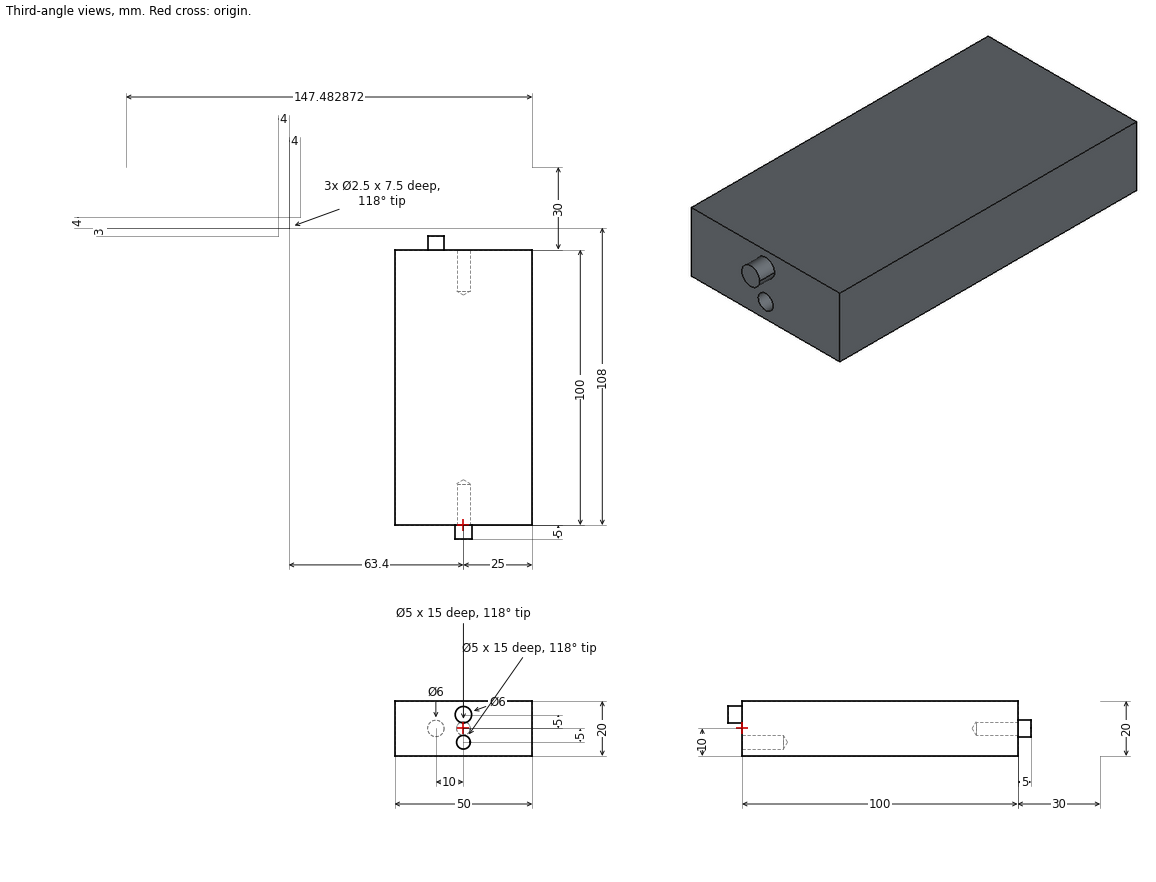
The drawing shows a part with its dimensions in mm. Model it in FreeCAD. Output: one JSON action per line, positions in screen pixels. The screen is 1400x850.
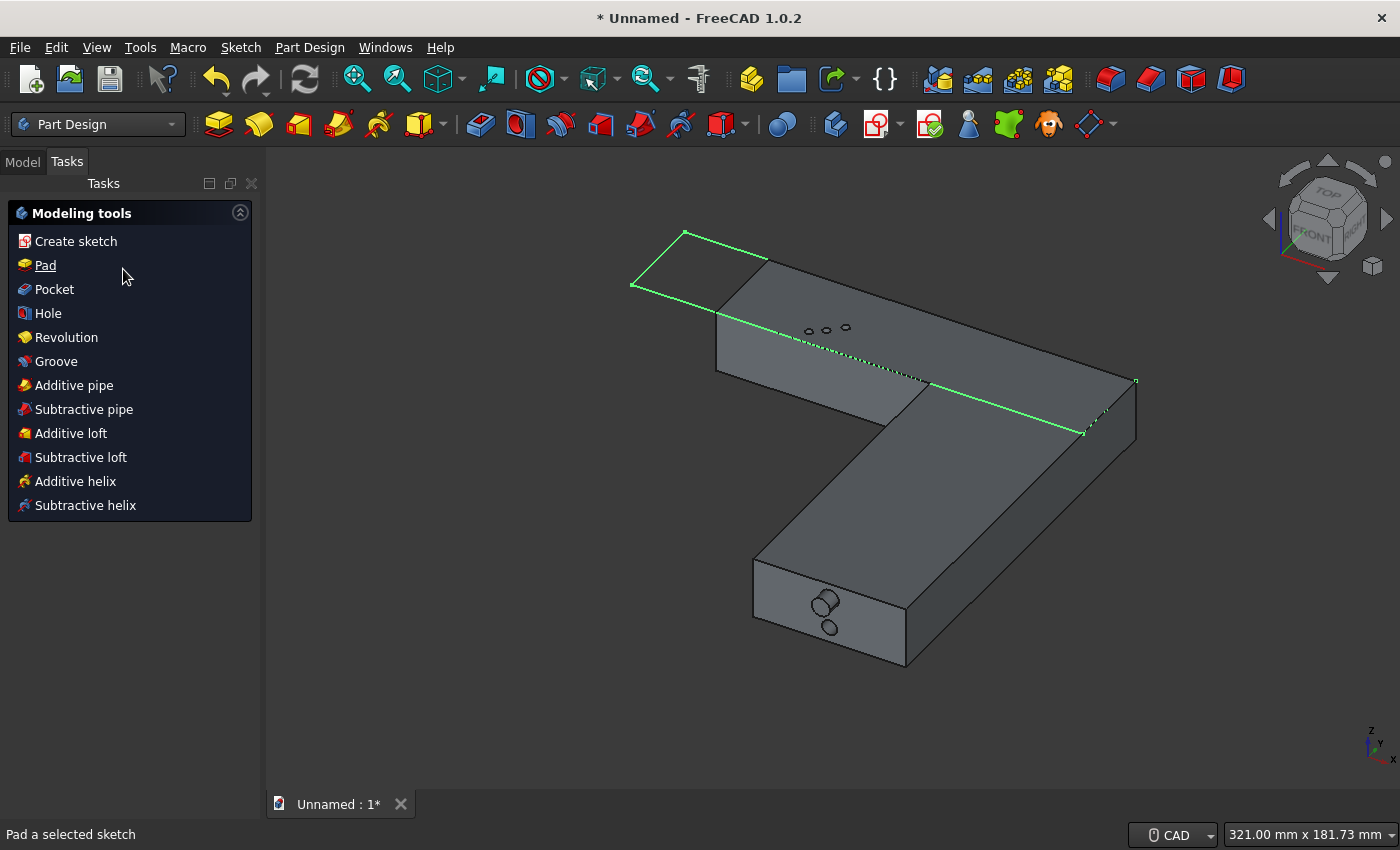
{"action": "left_click", "coordinate": [482, 124]}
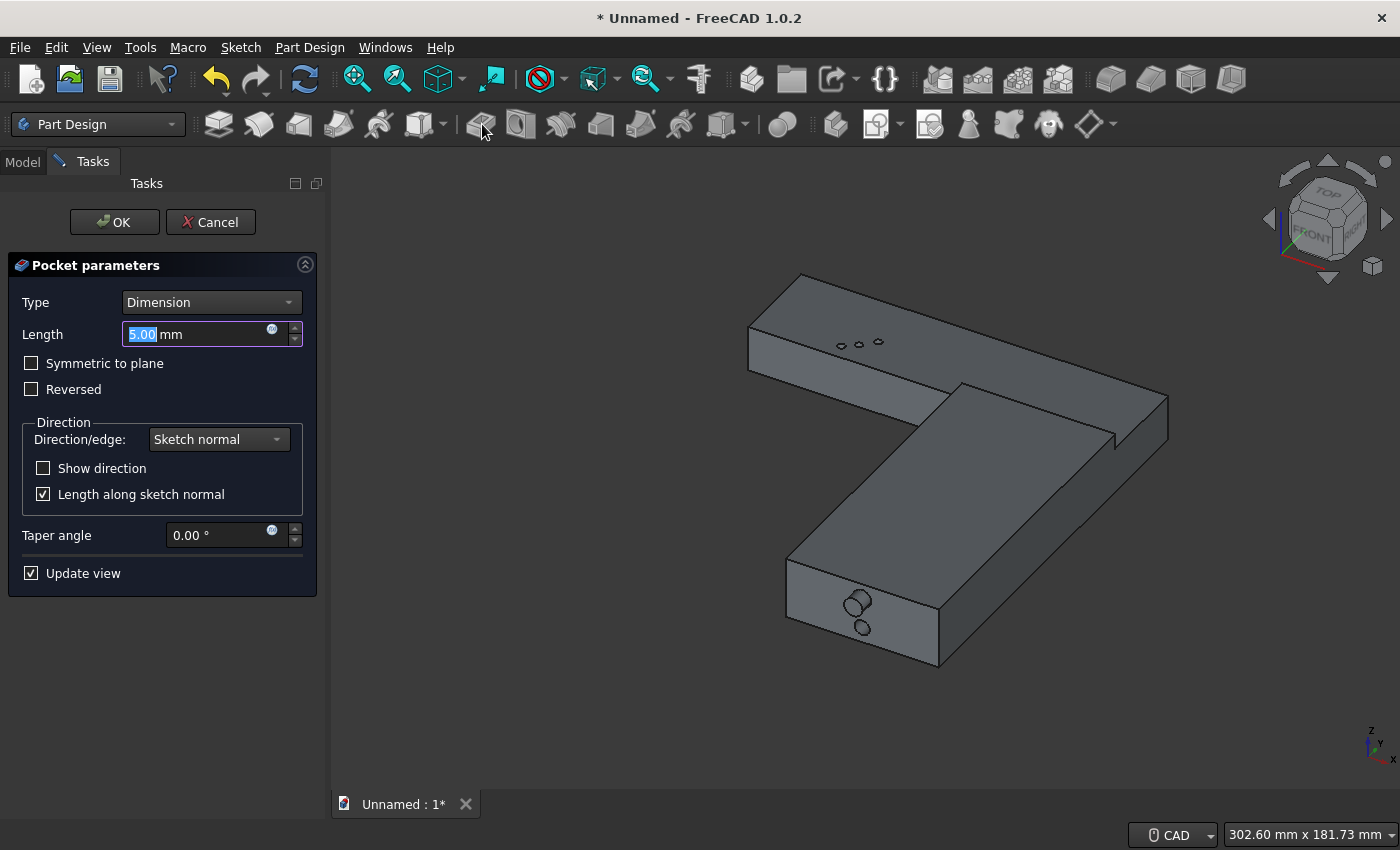
{"action": "left_click", "coordinate": [212, 302]}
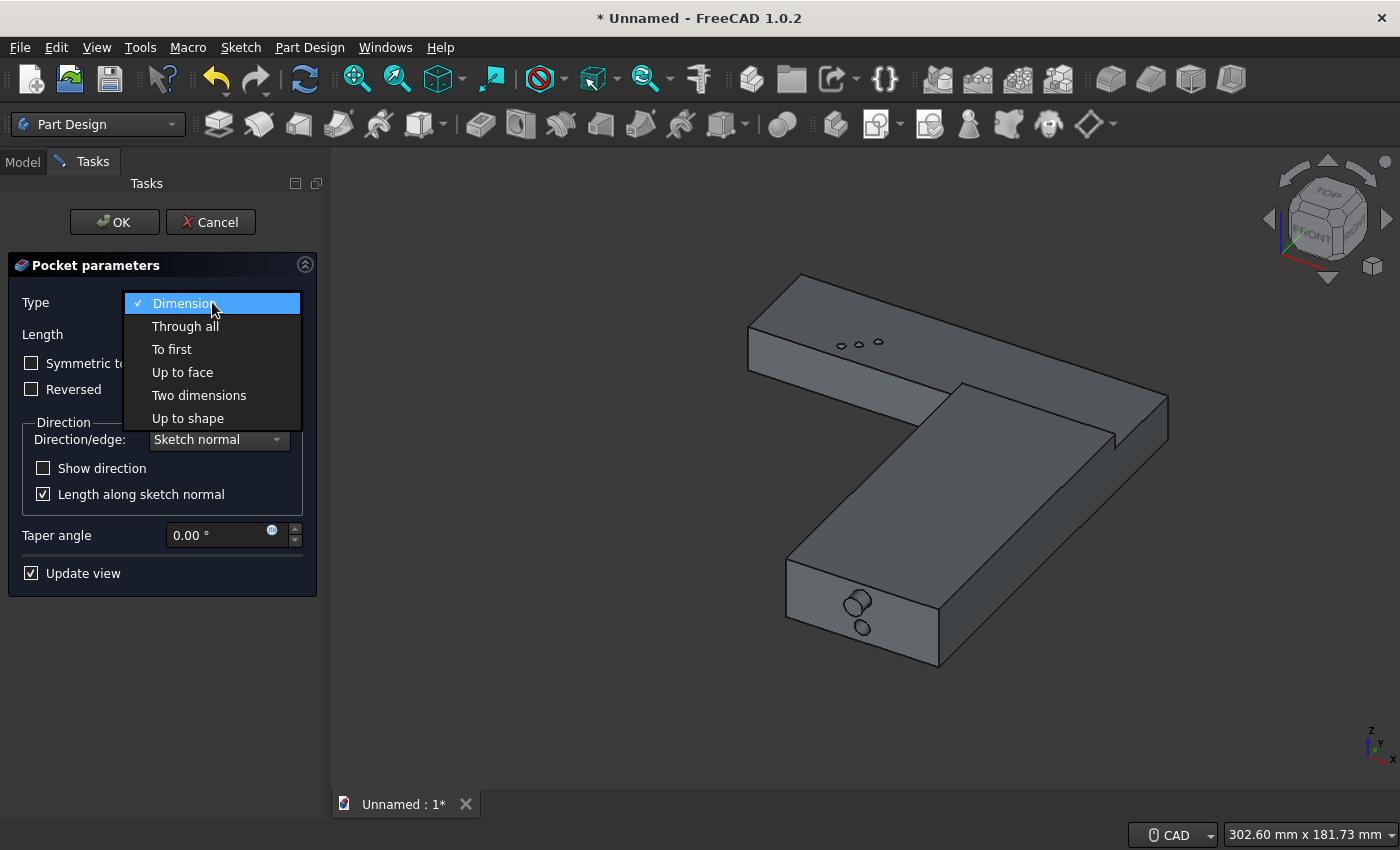
{"action": "left_click", "coordinate": [212, 326]}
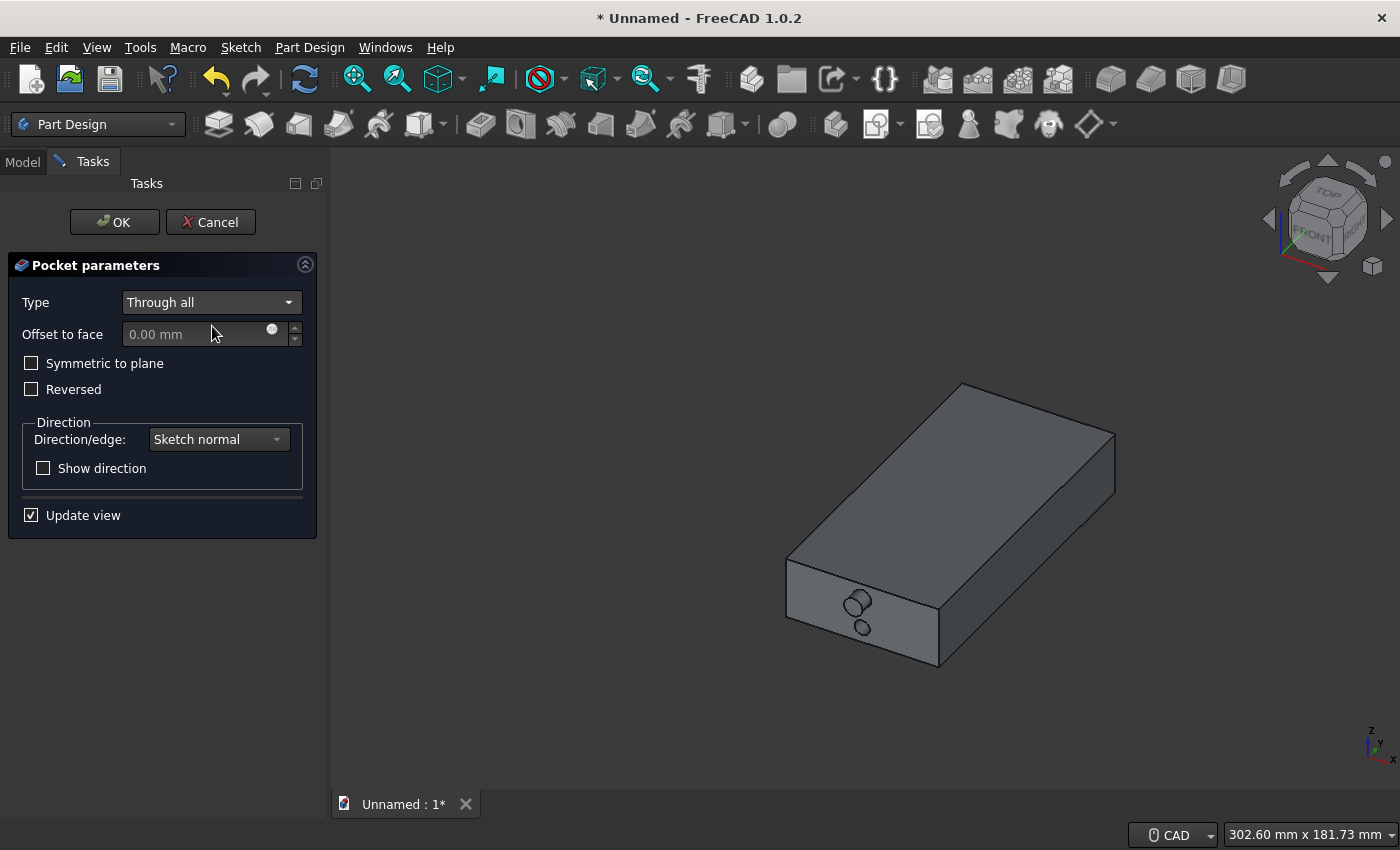
{"action": "left_click", "coordinate": [115, 222]}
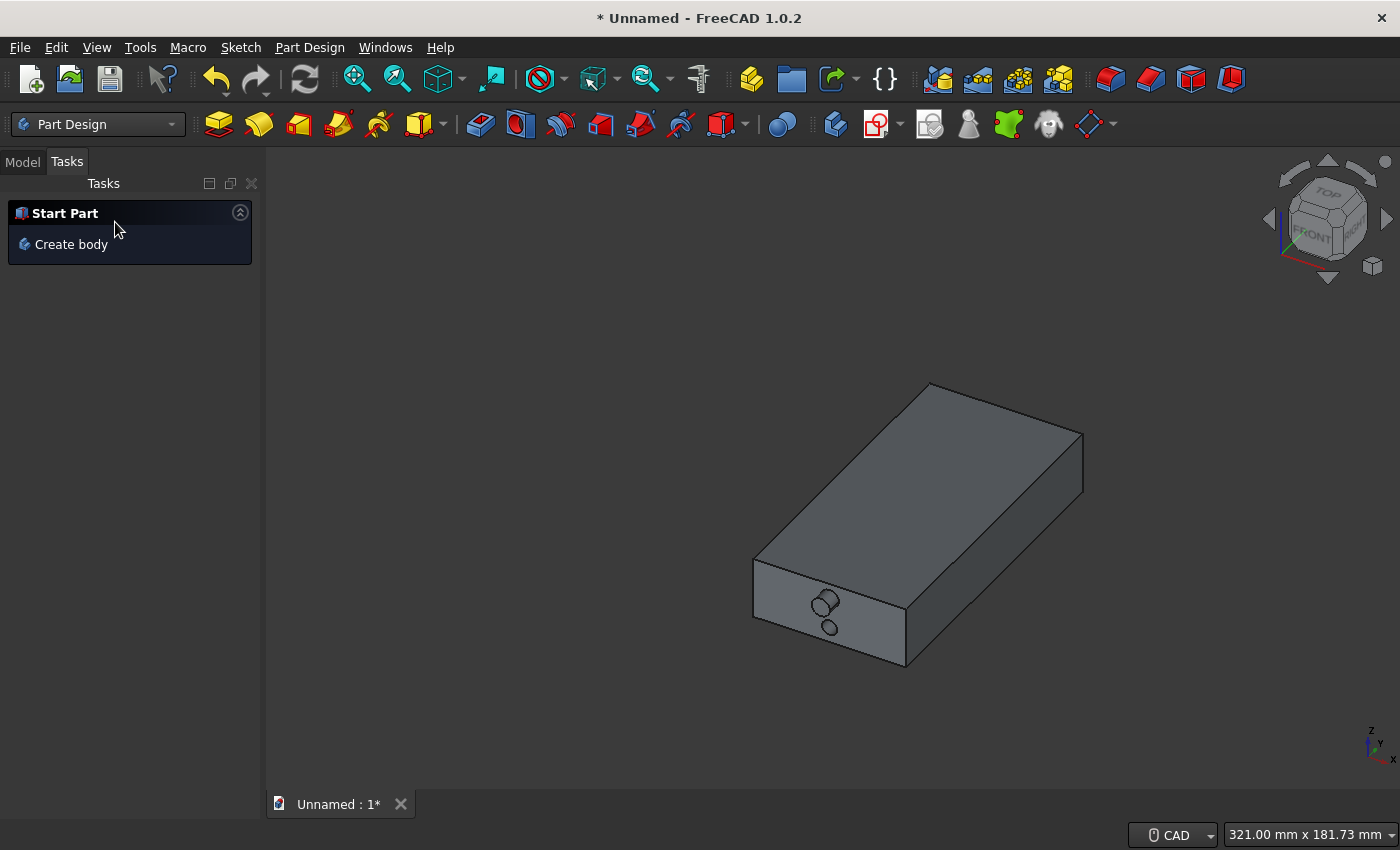
{"action": "key", "text": "4"}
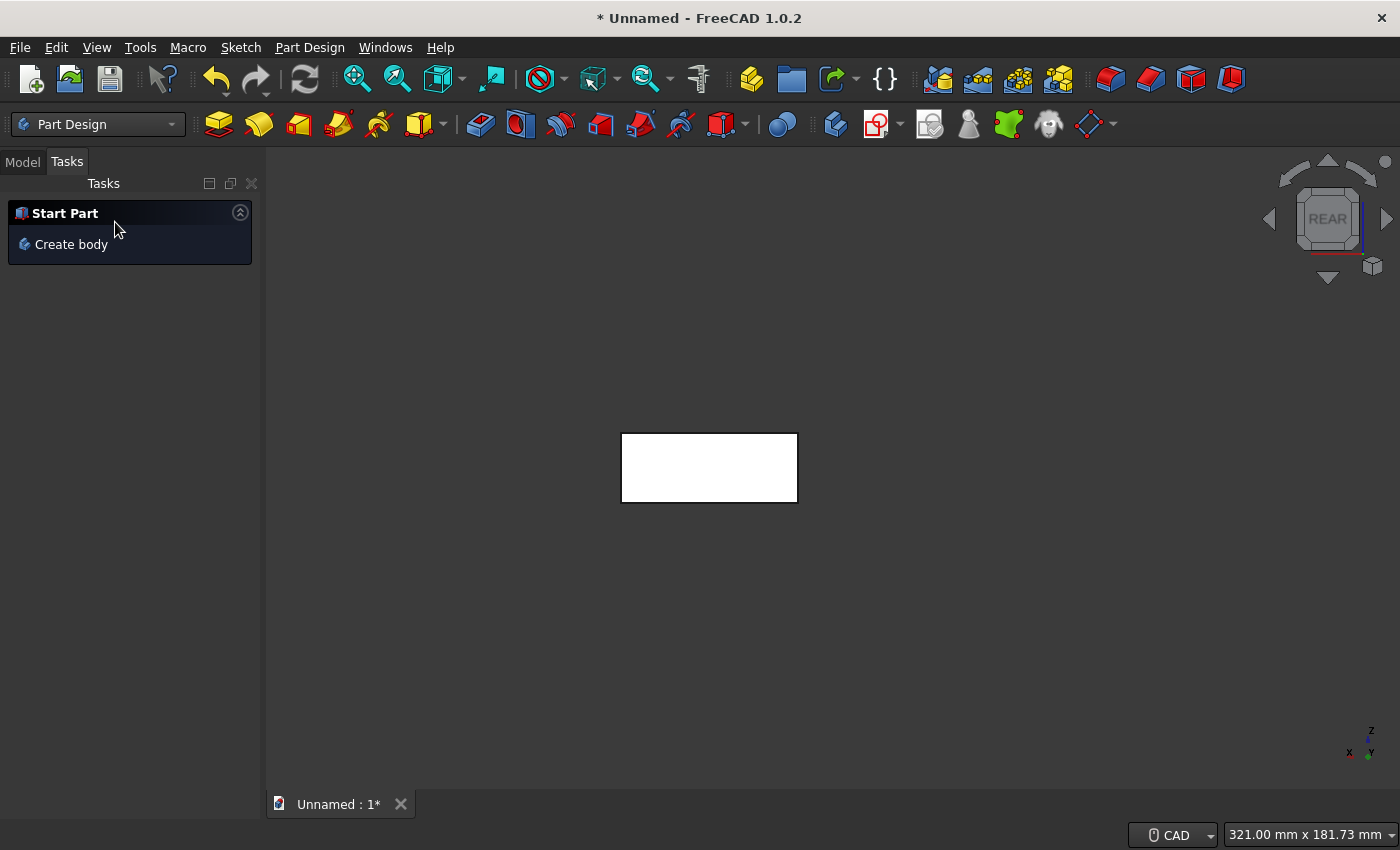
{"action": "left_click", "coordinate": [358, 80]}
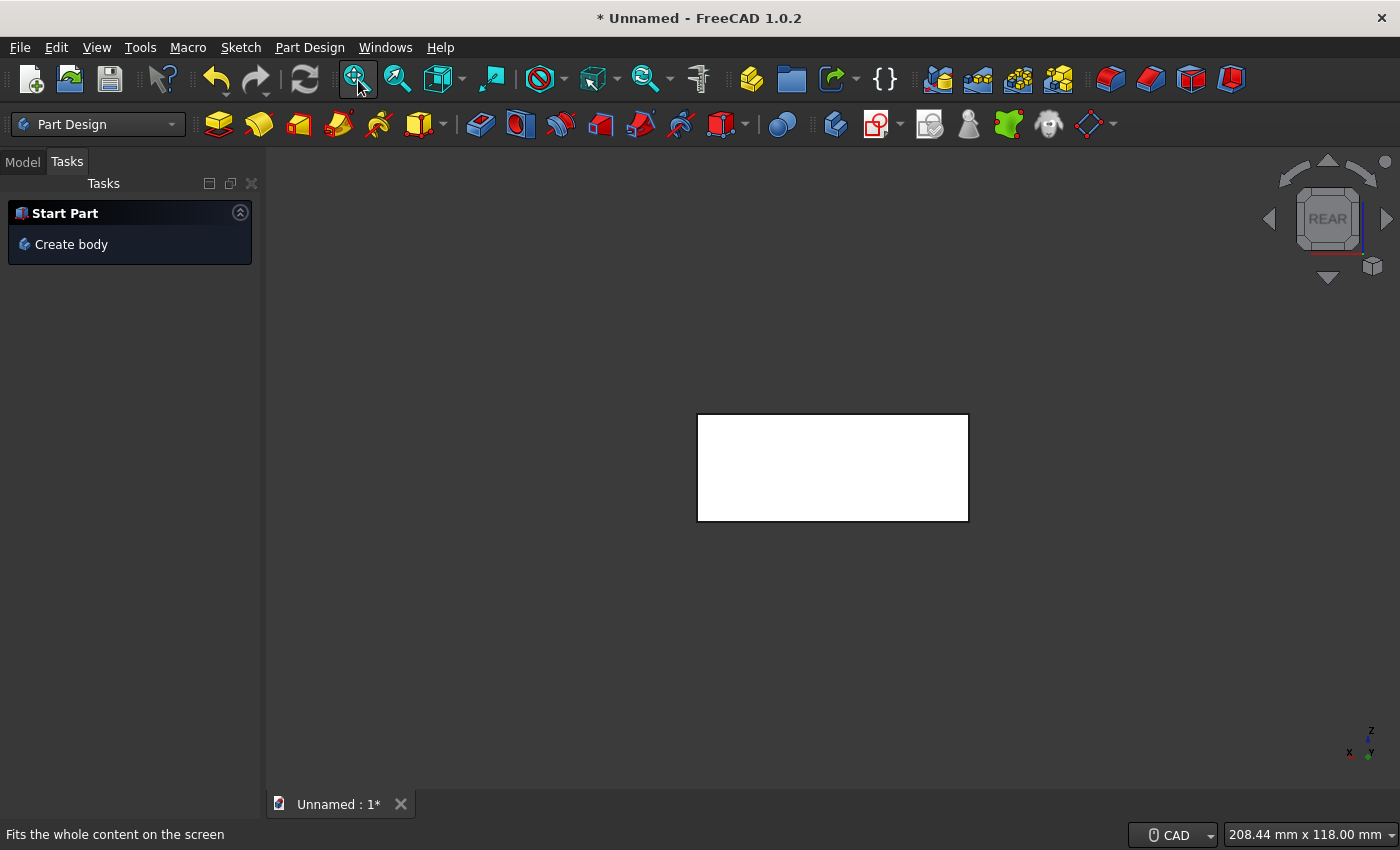
{"action": "left_click", "coordinate": [755, 467]}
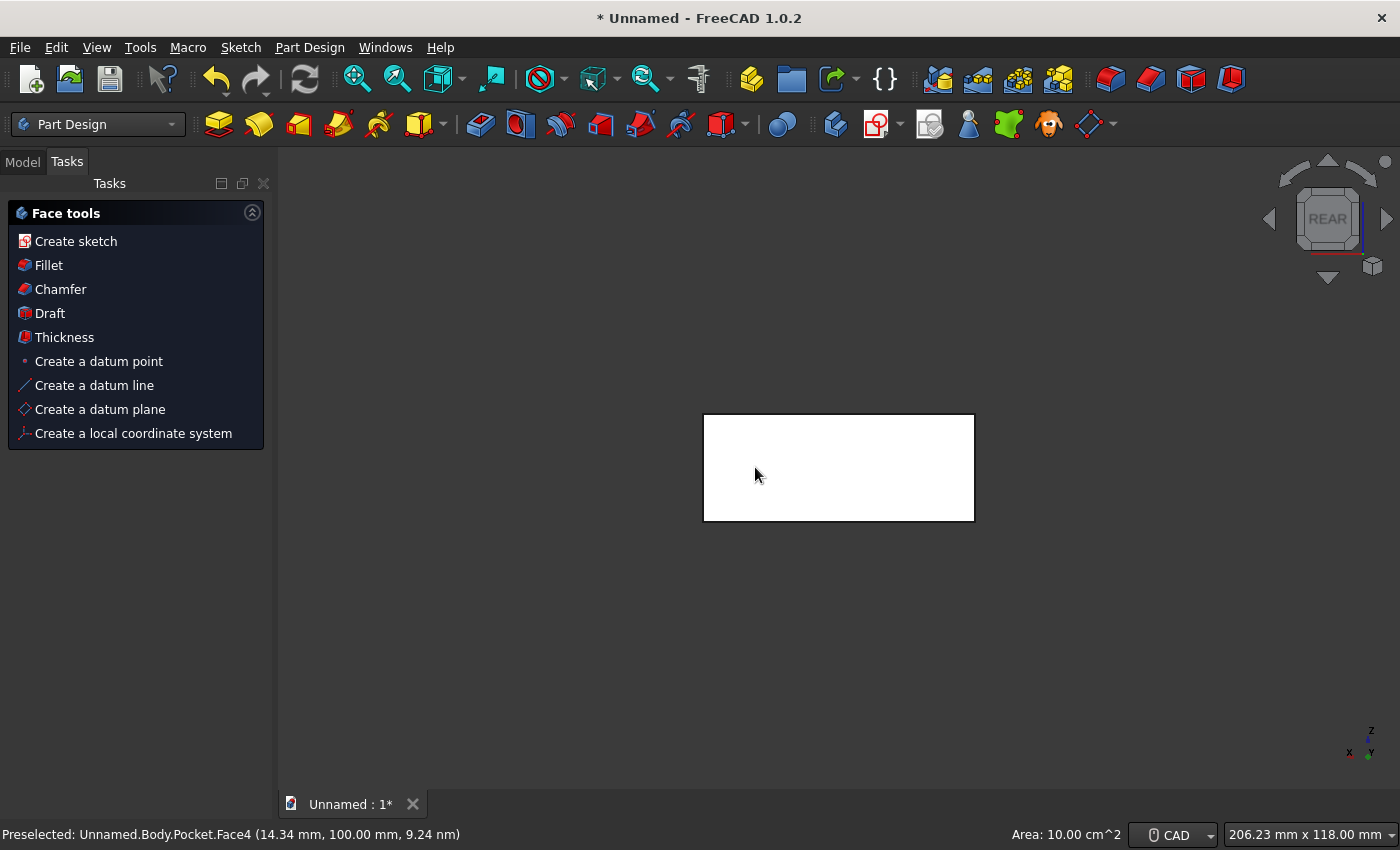
{"action": "left_click", "coordinate": [876, 124]}